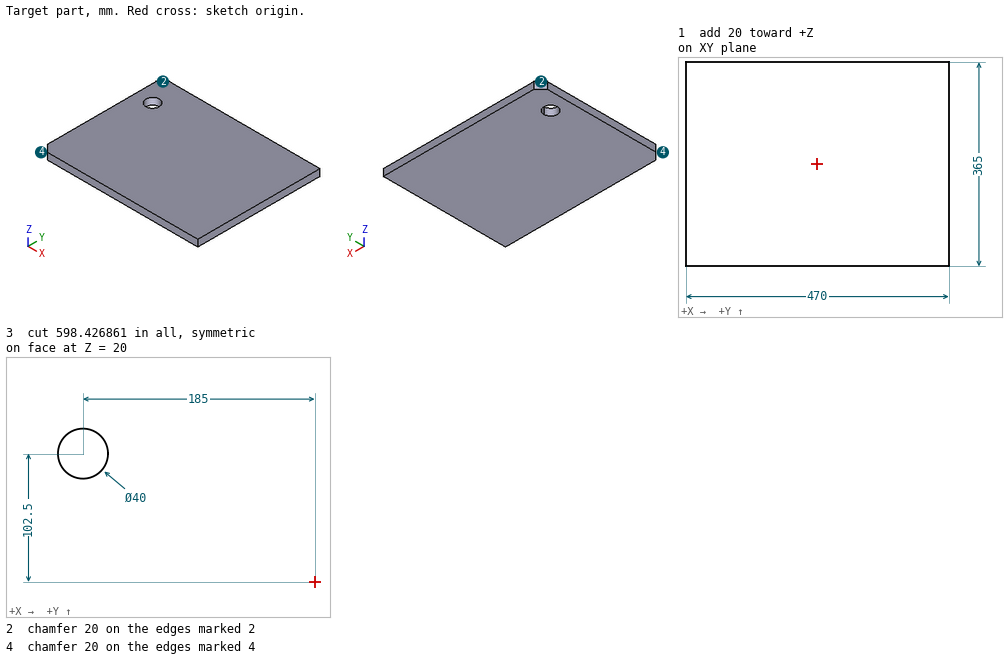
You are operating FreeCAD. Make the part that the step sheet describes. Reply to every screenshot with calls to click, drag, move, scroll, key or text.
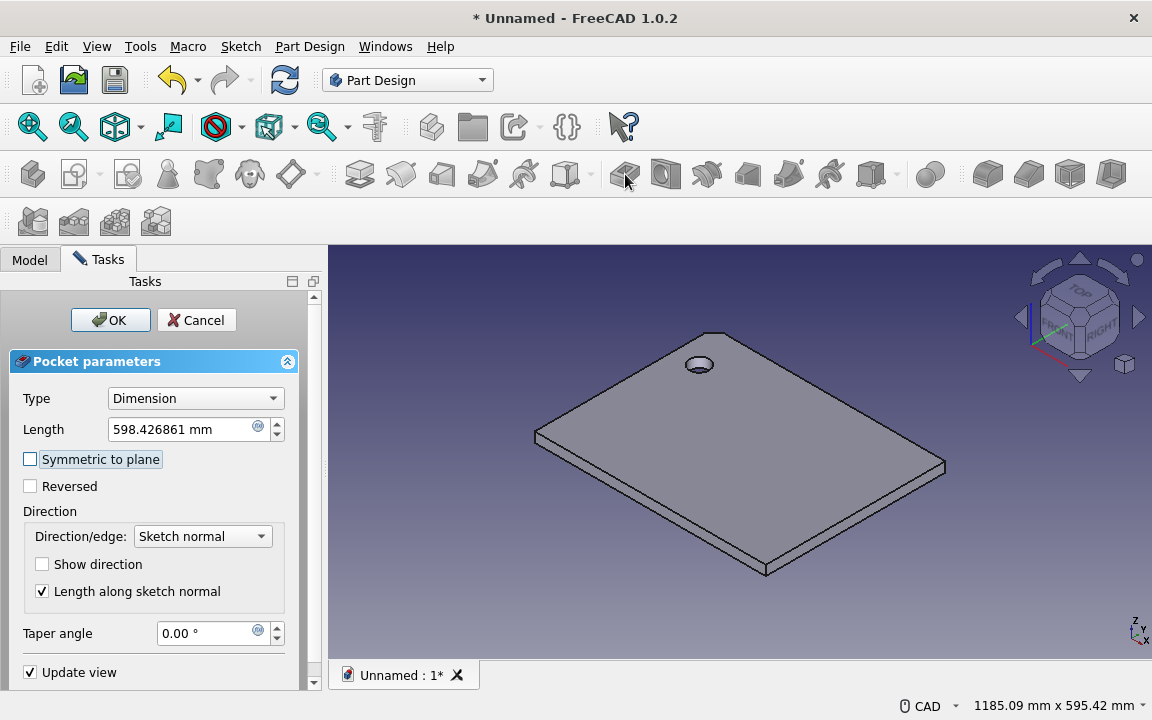
click(31, 459)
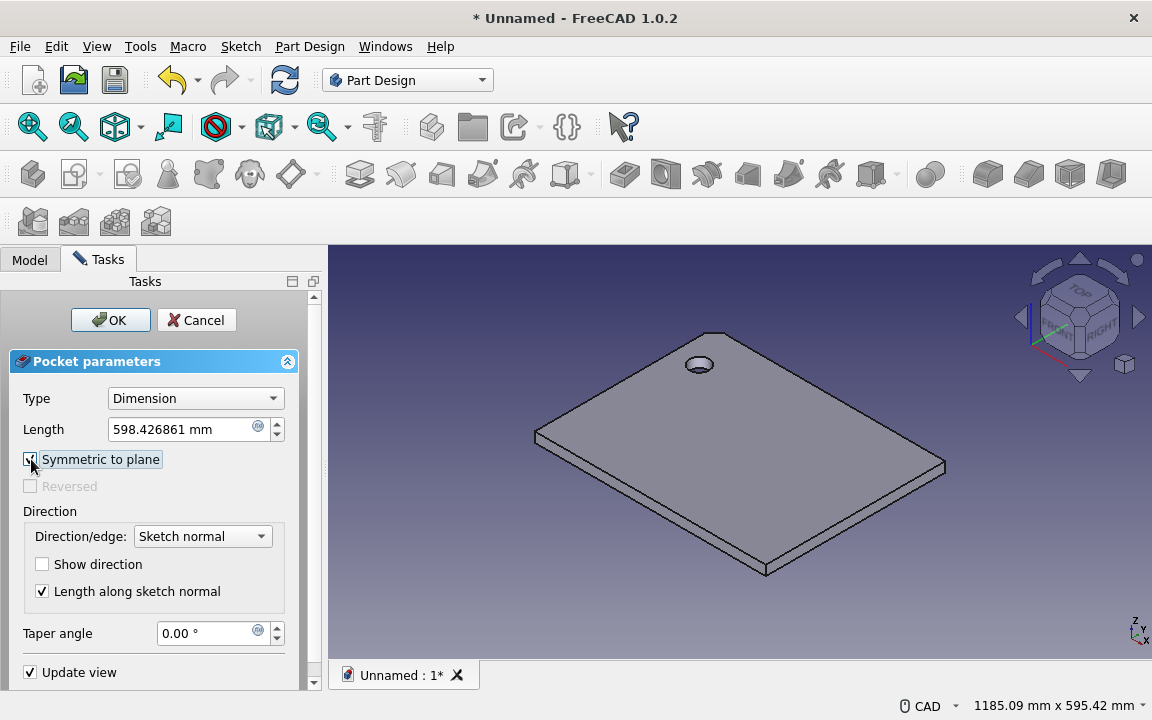
click(111, 320)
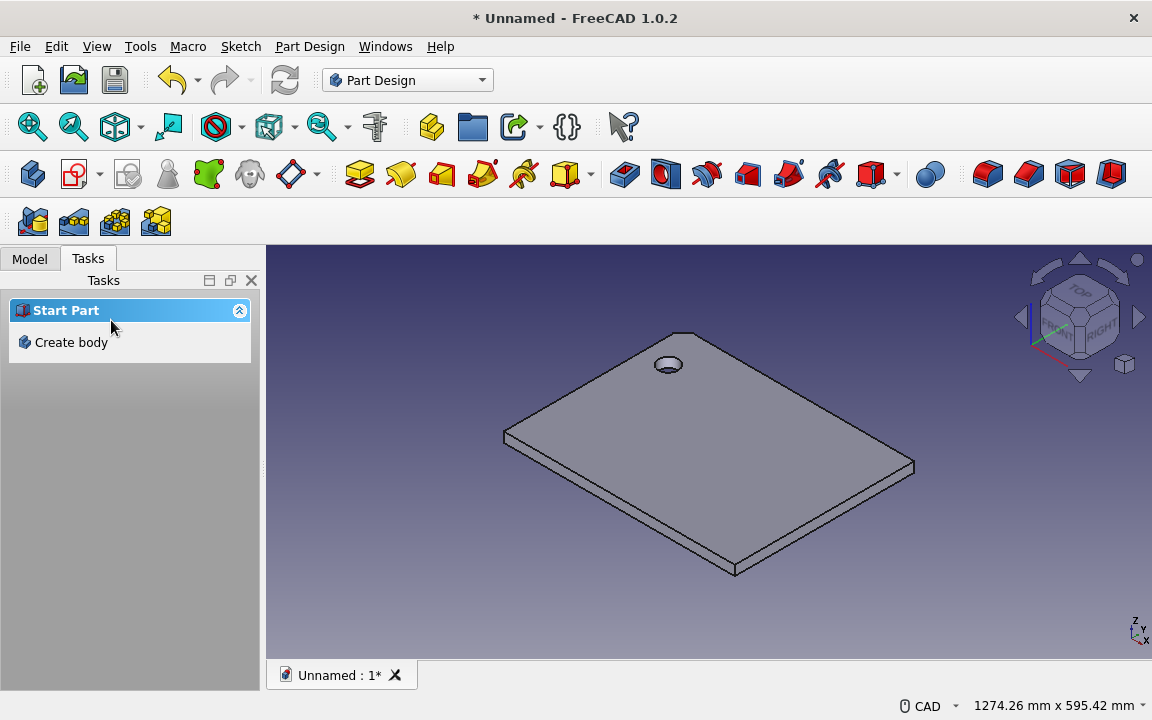
scroll(504, 436, up, 6)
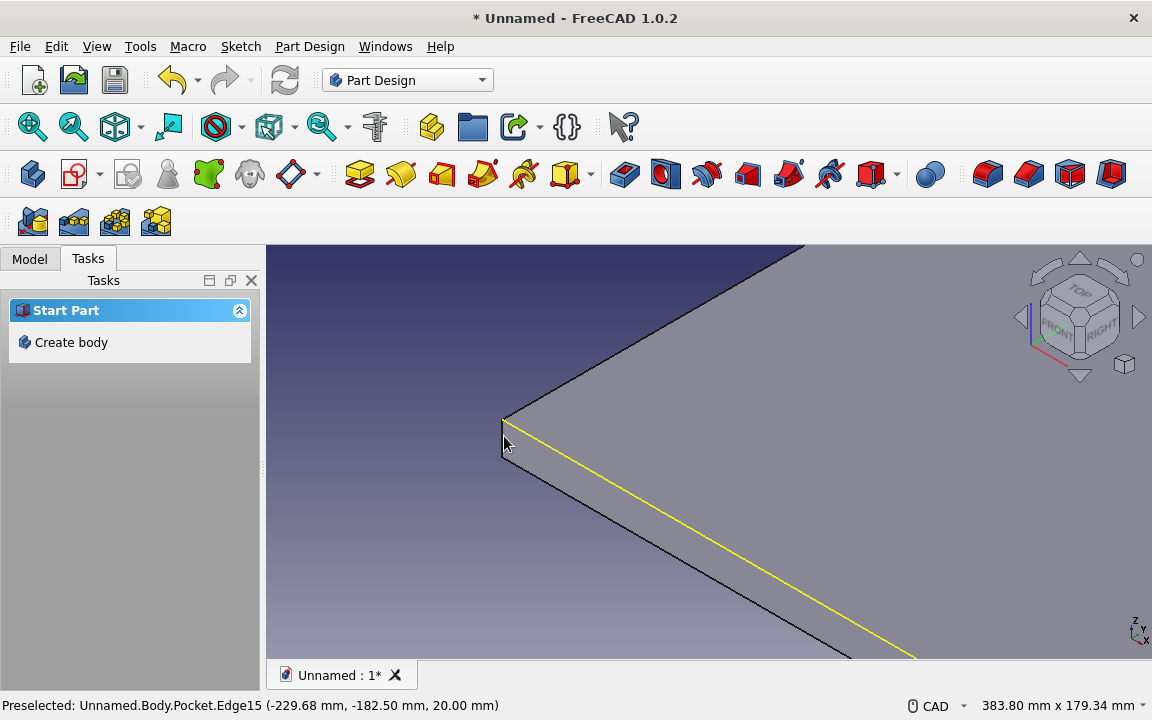
click(33, 128)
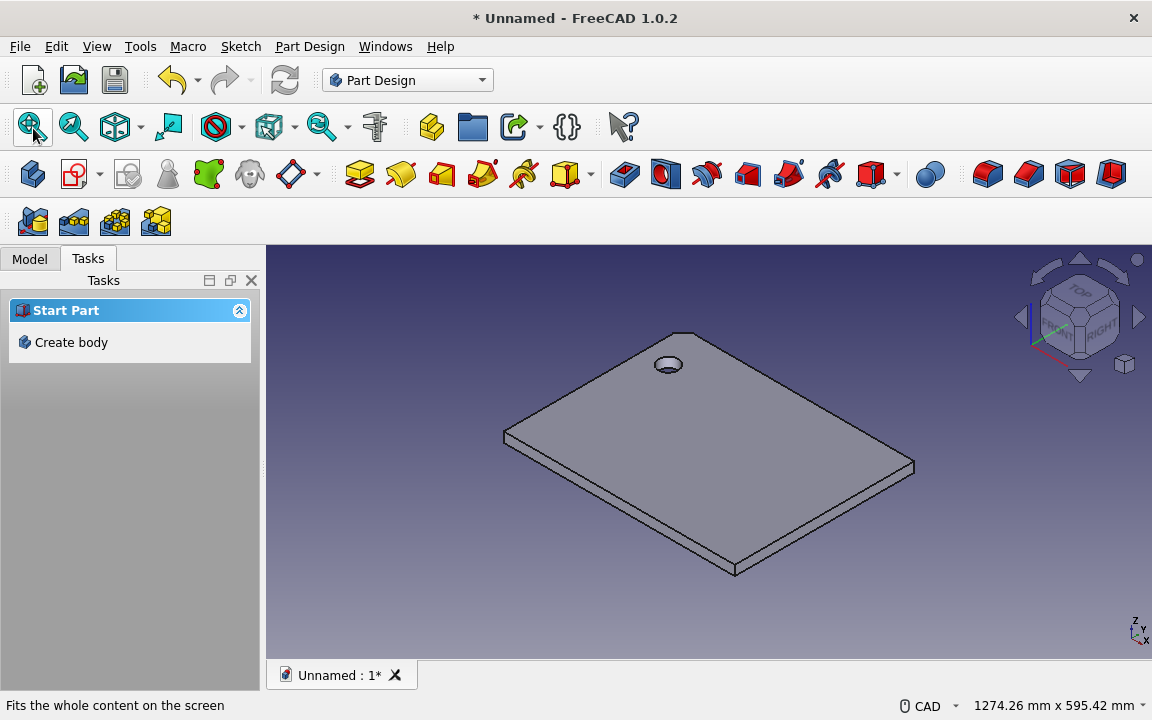
key(2)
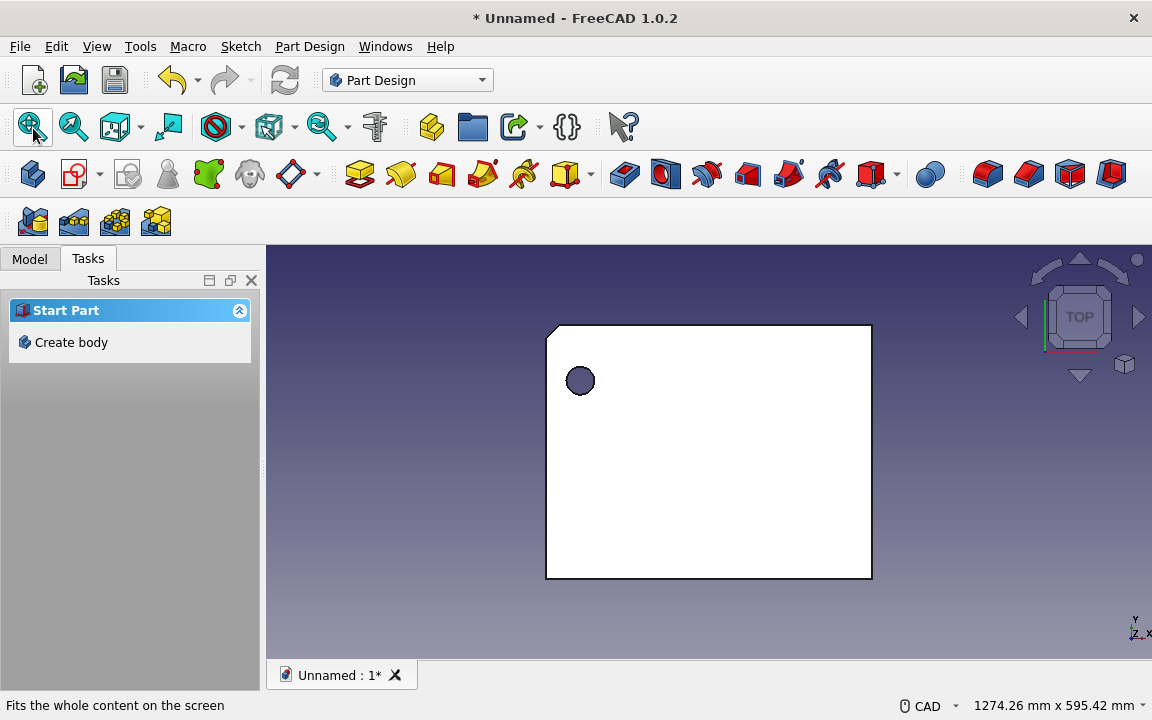
scroll(546, 578, up, 6)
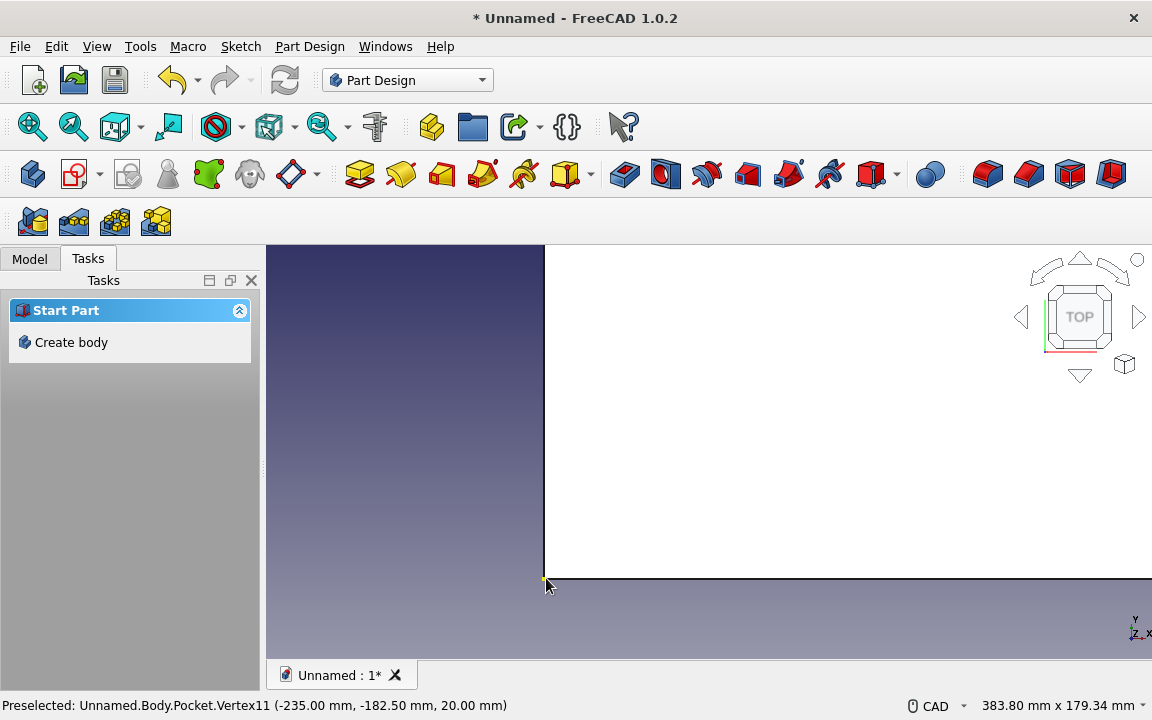
click(33, 128)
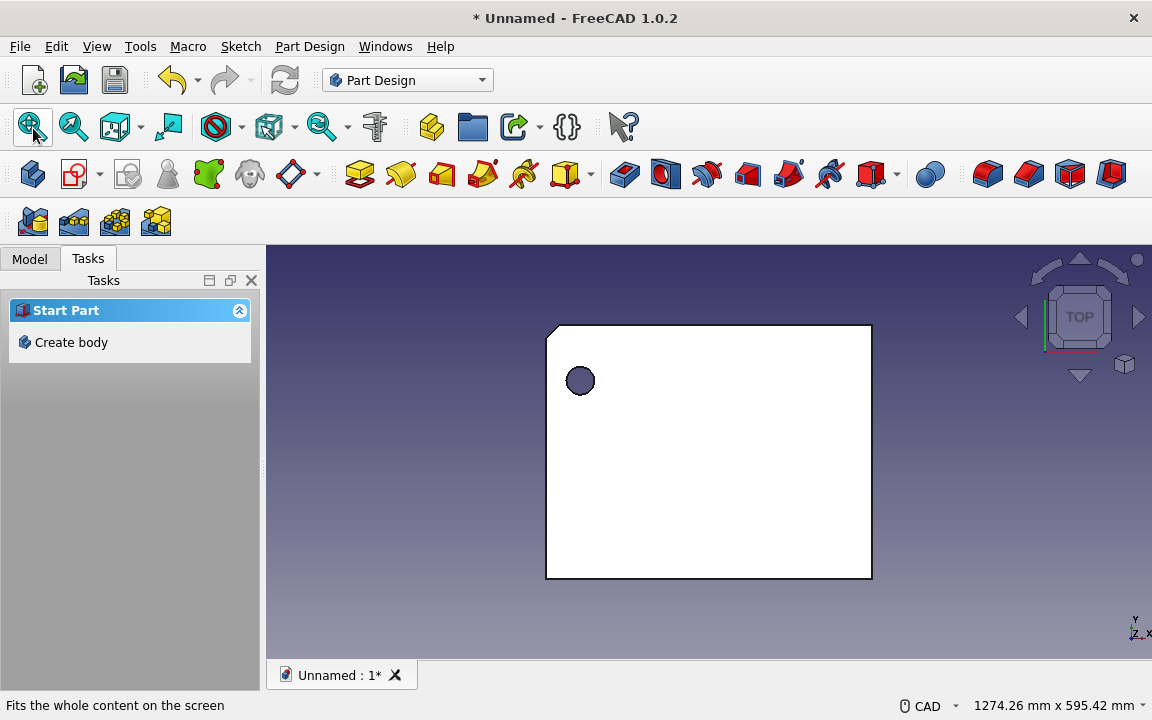
key(0)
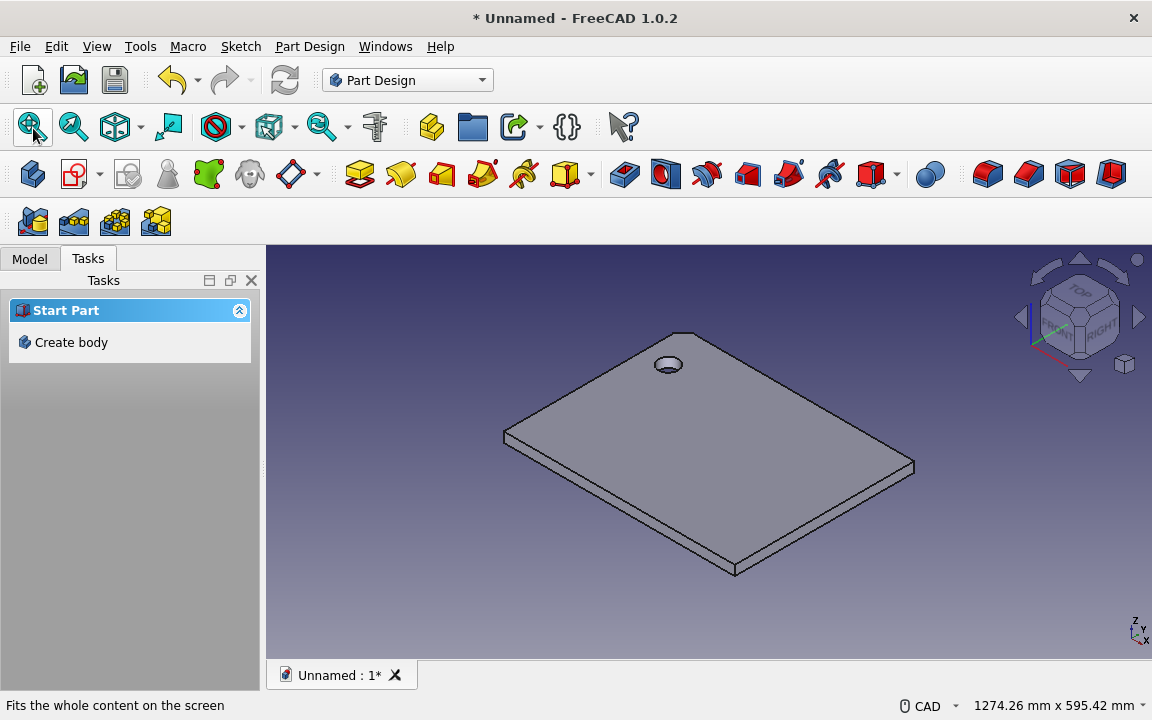
scroll(504, 436, up, 6)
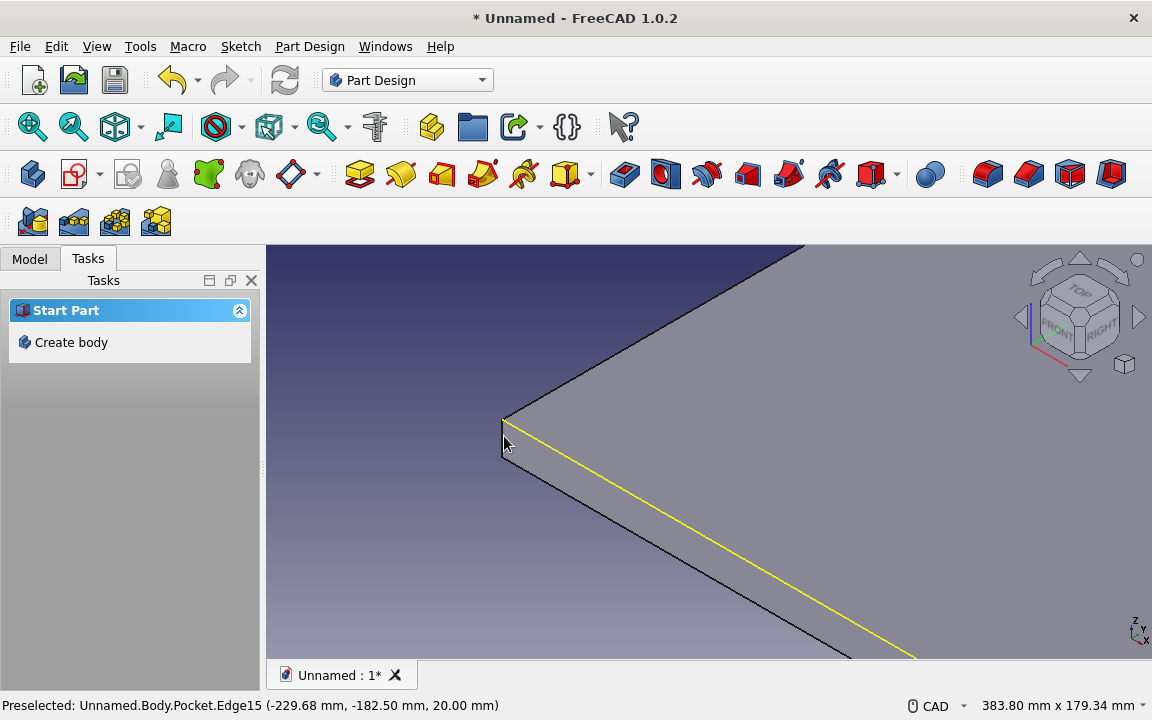
click(33, 128)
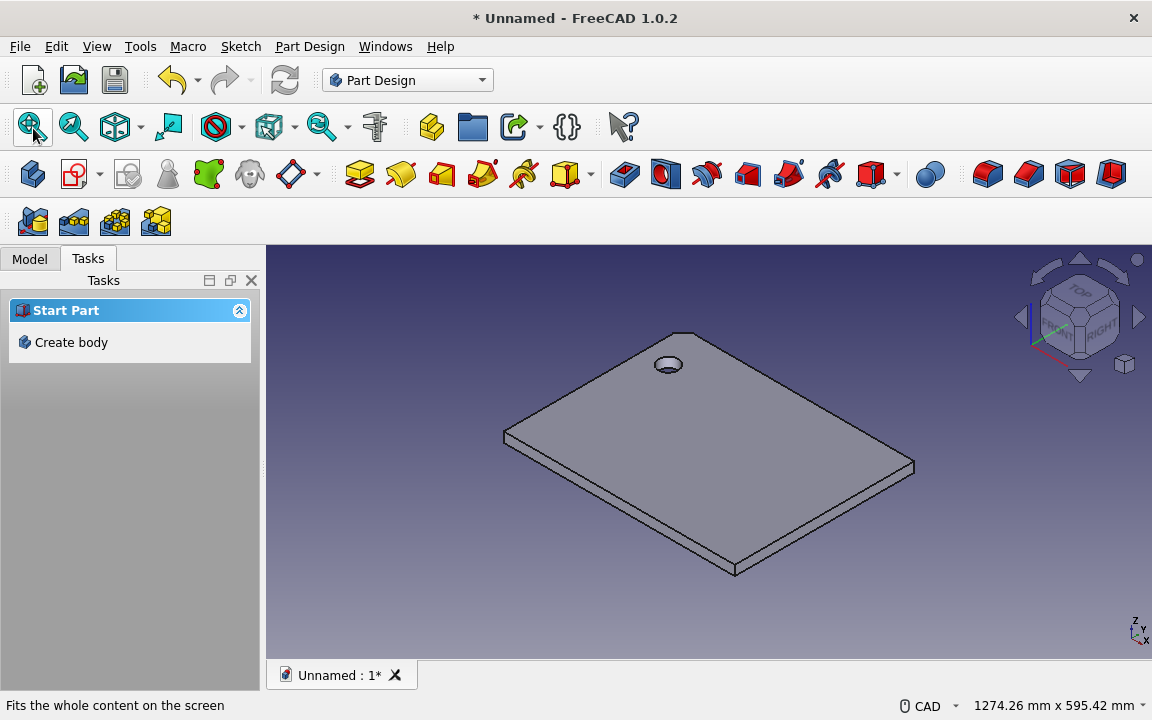
key(1)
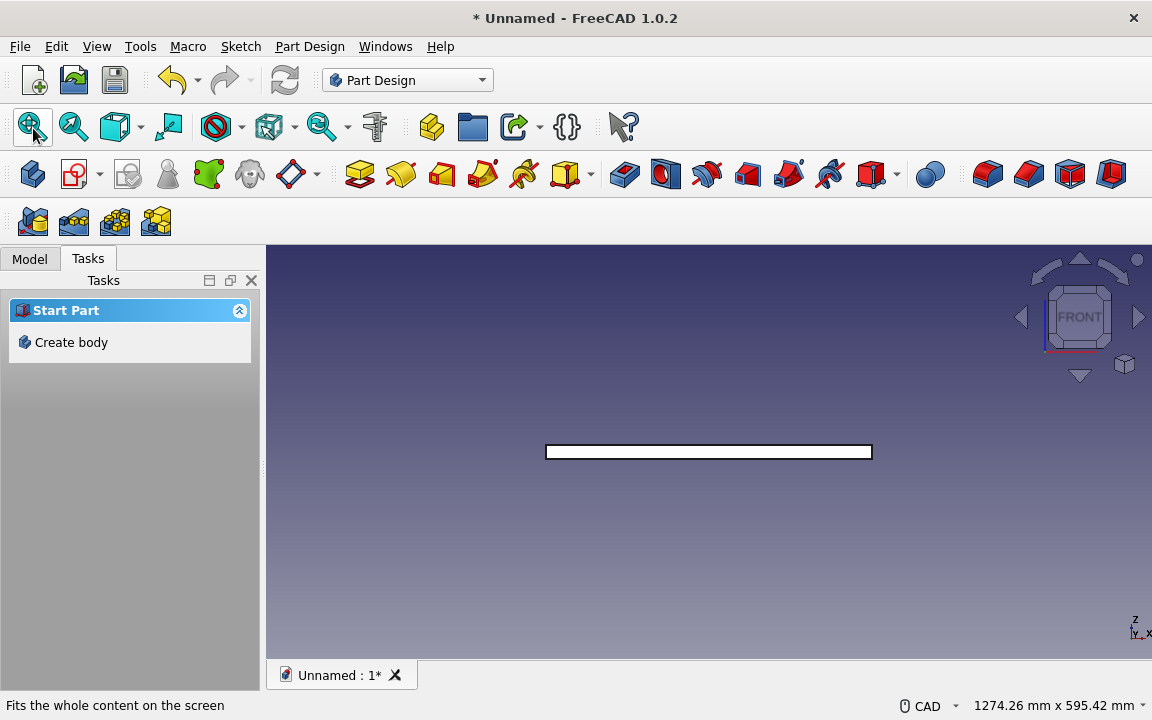
click(33, 128)